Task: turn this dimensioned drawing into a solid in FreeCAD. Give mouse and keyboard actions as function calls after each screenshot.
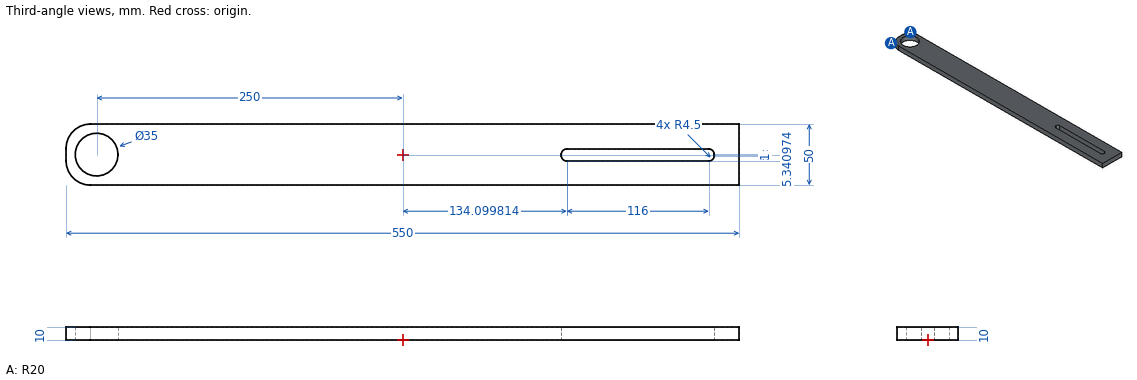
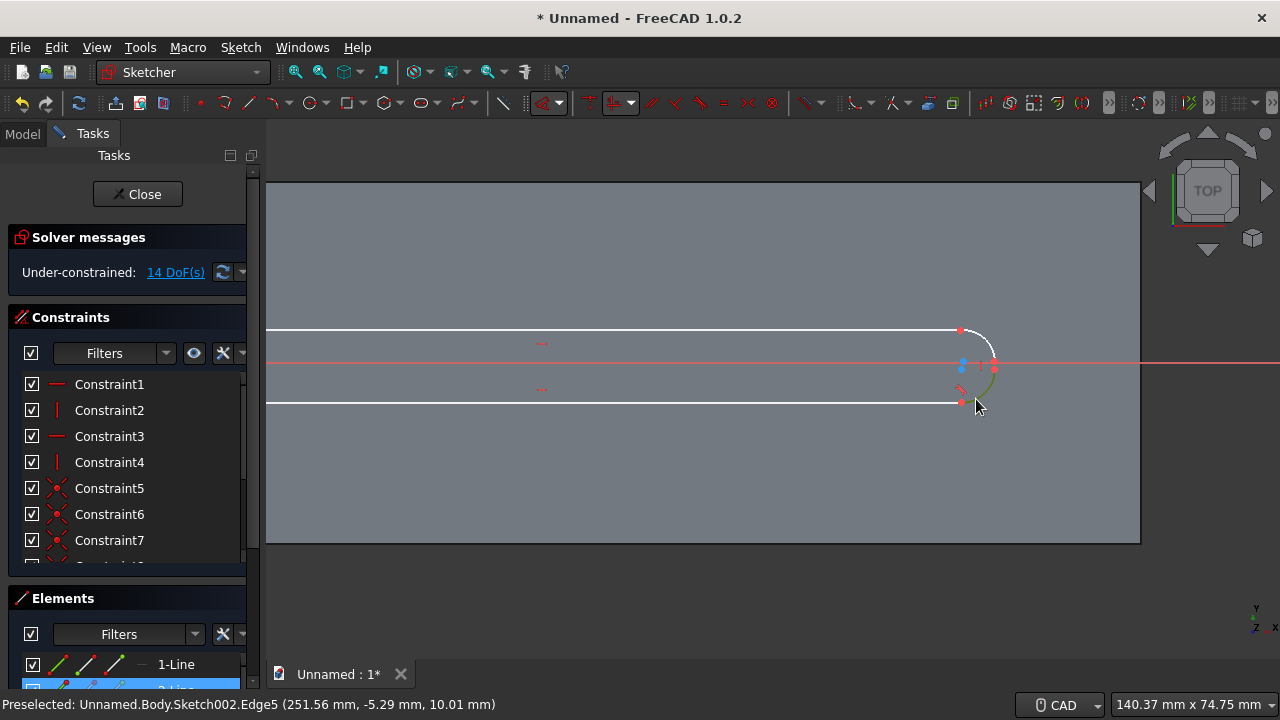
click(700, 104)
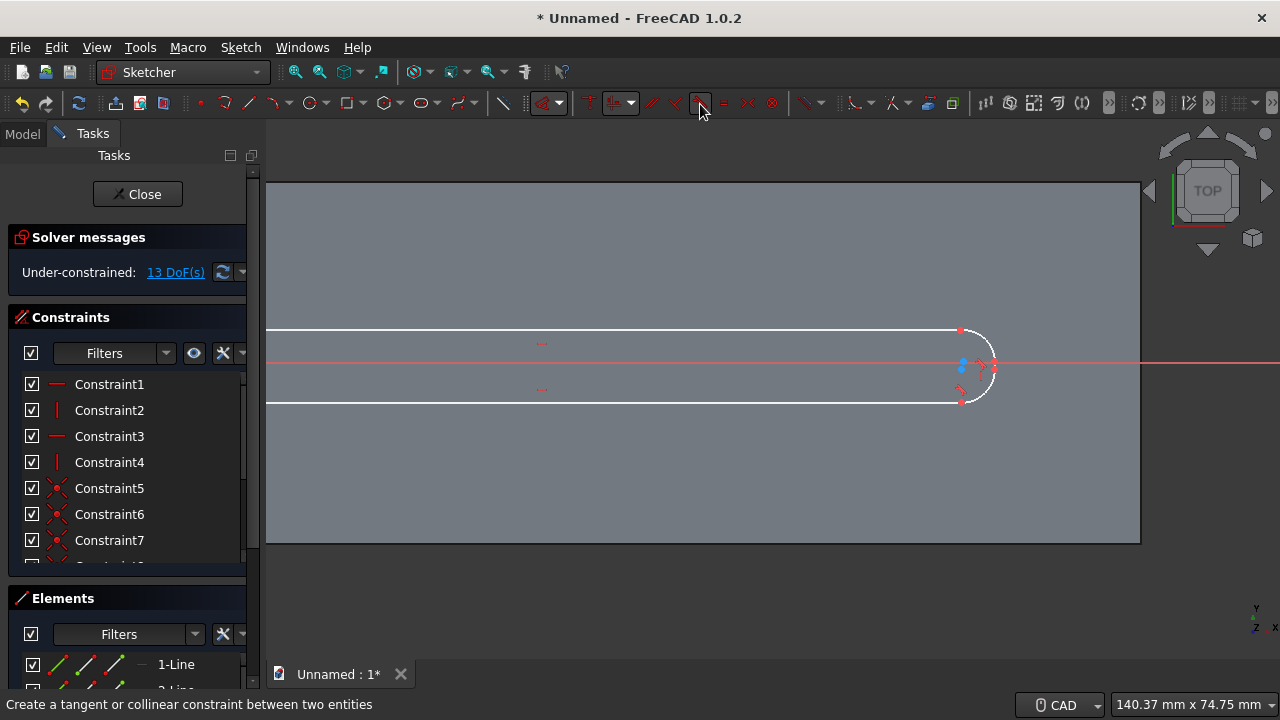
scroll(995, 366, up, 7)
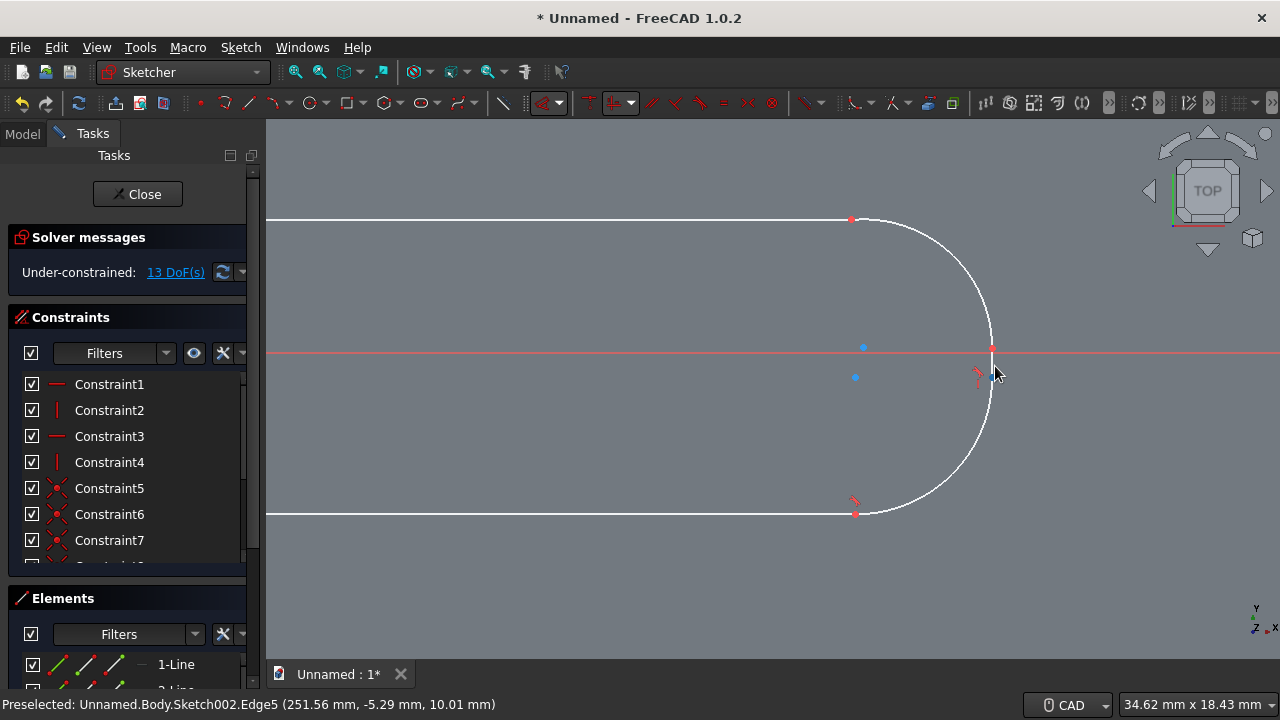
click(992, 363)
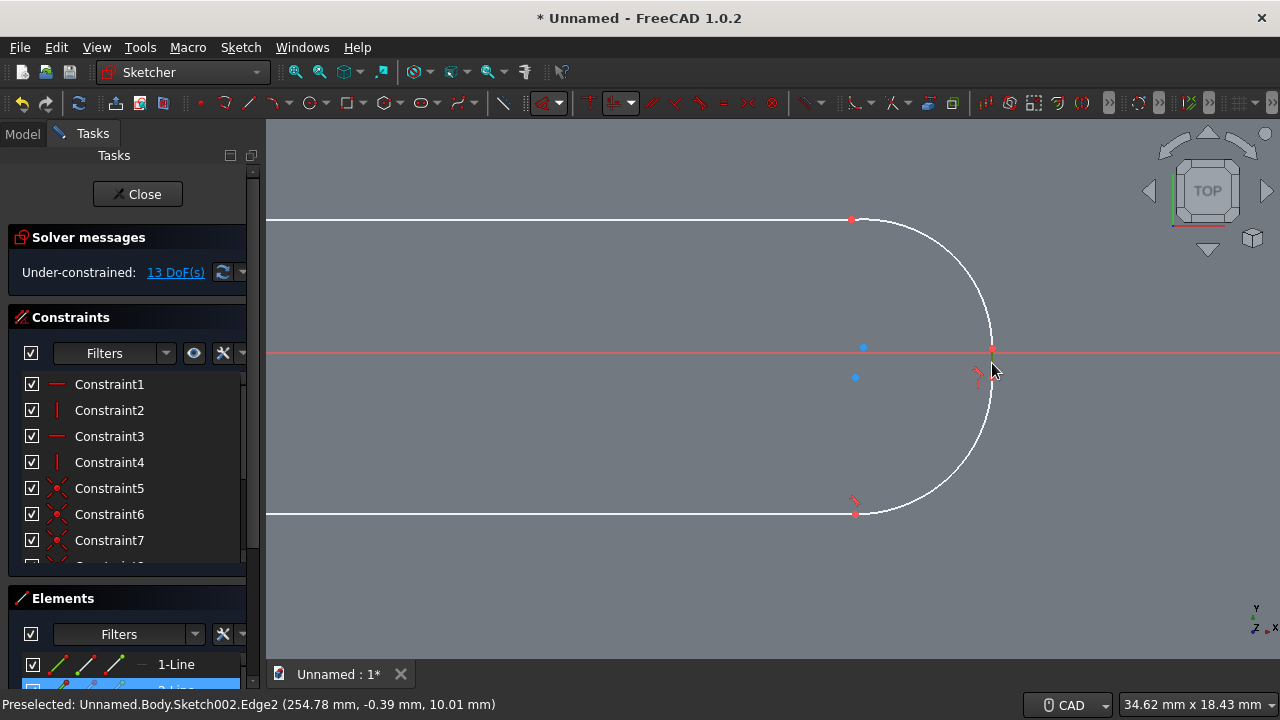
scroll(981, 391, down, 13)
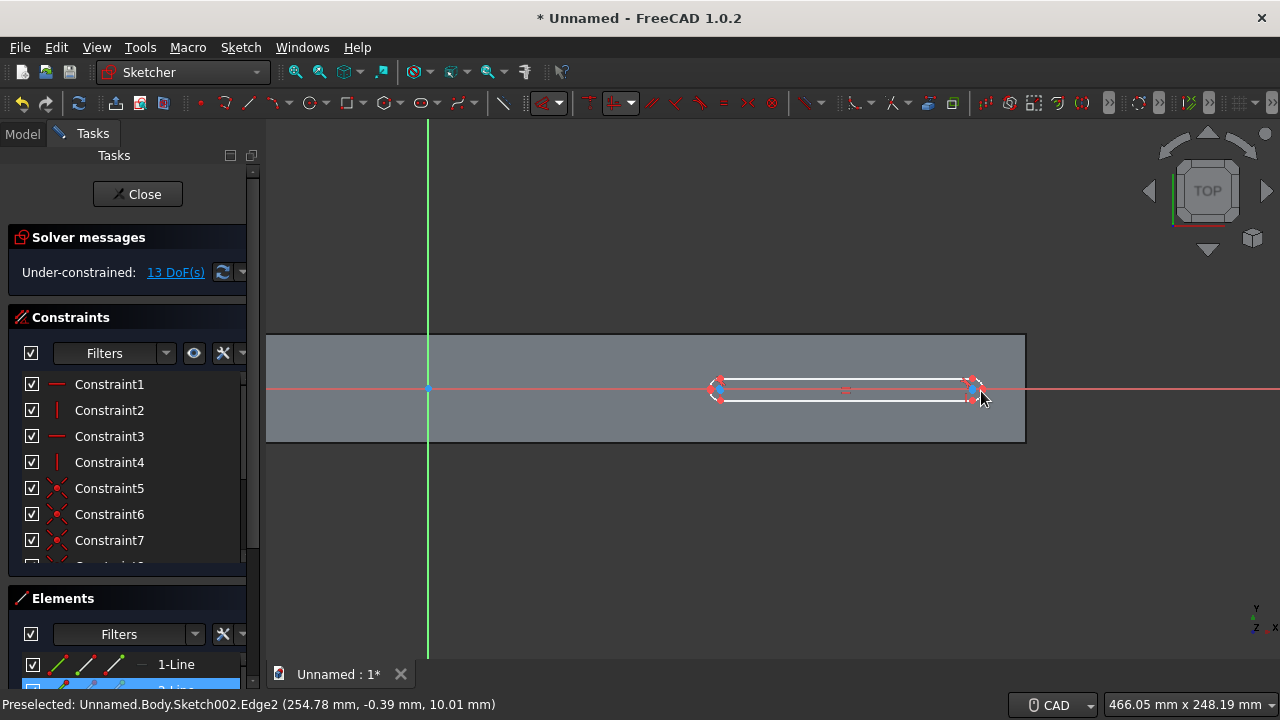
scroll(981, 384, up, 6)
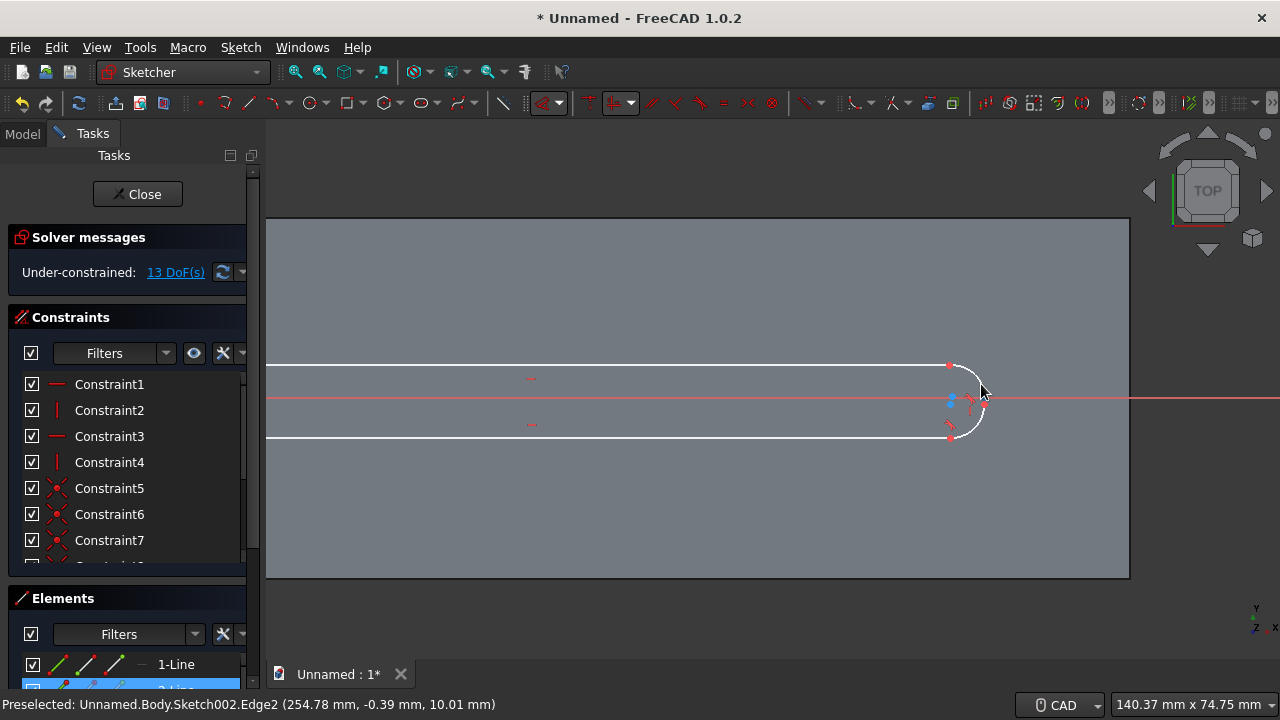
click(980, 382)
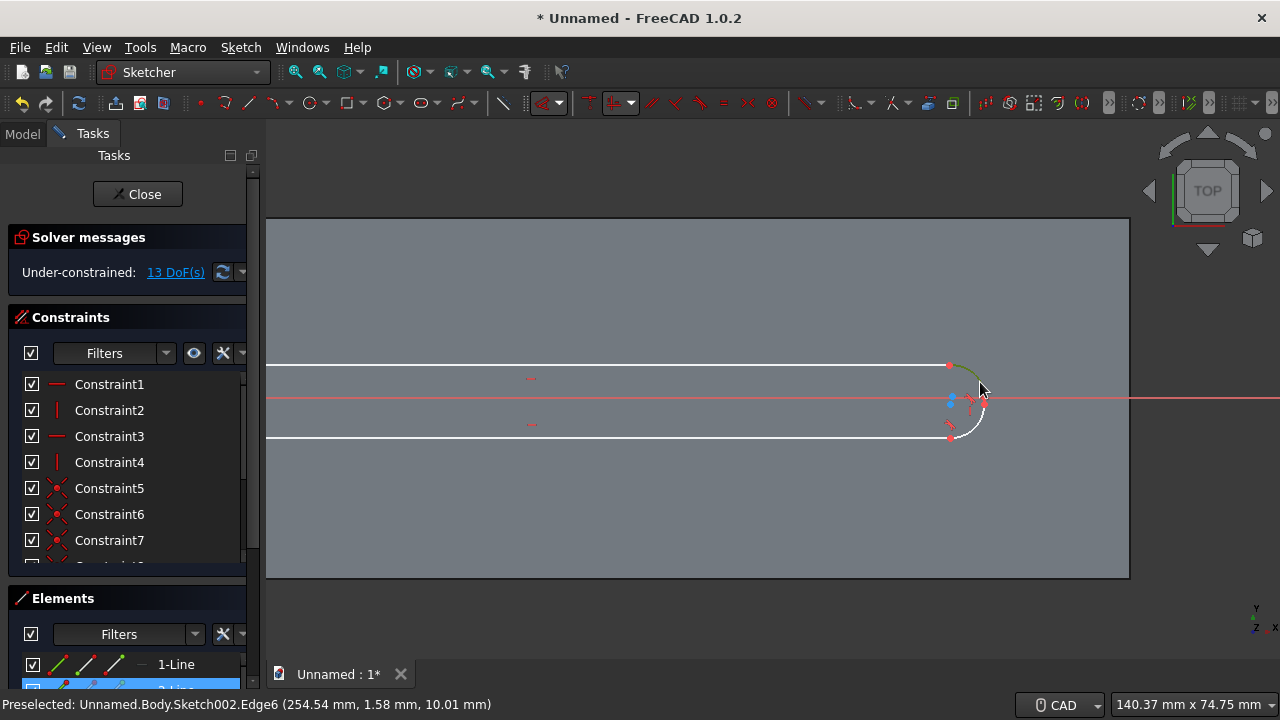
click(700, 104)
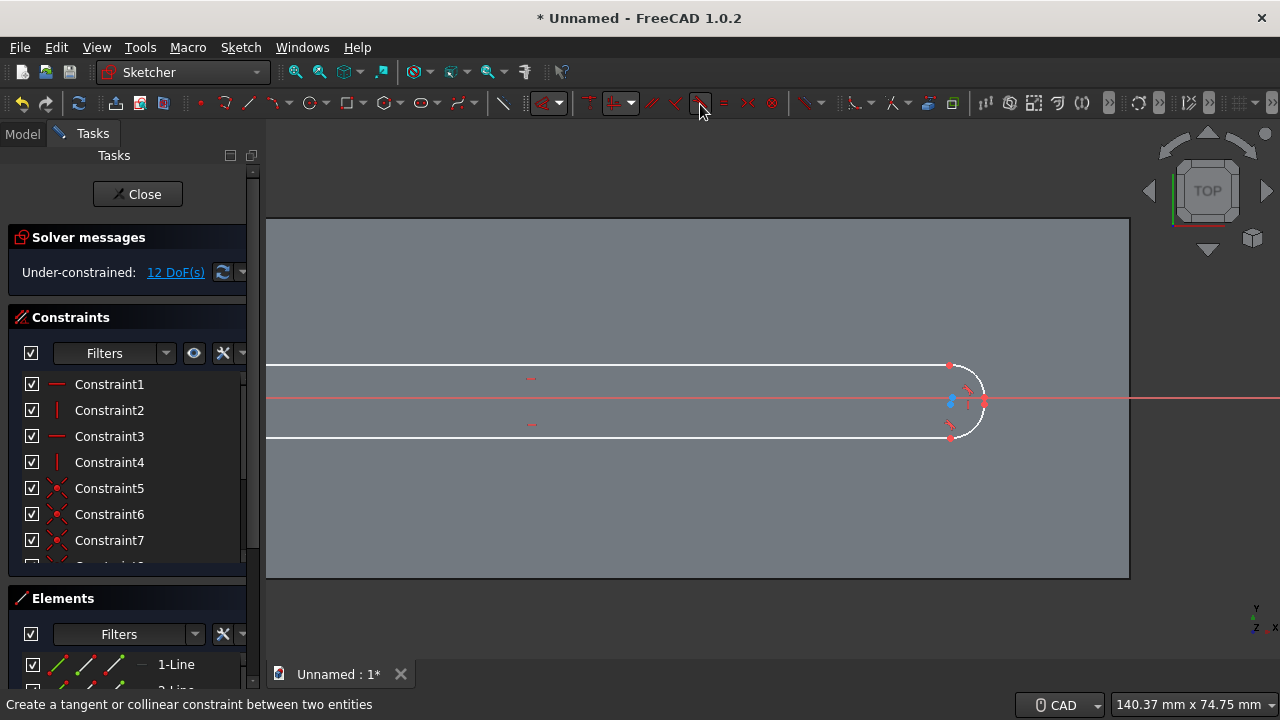
click(699, 365)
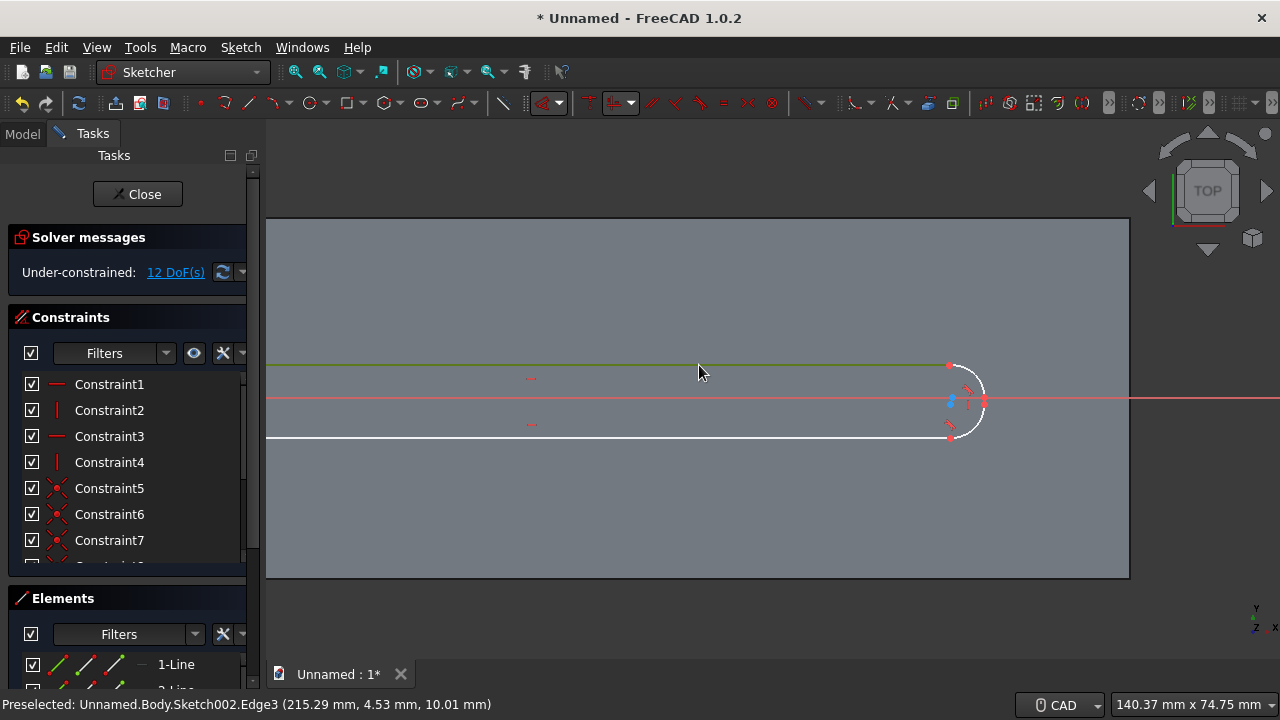
click(980, 382)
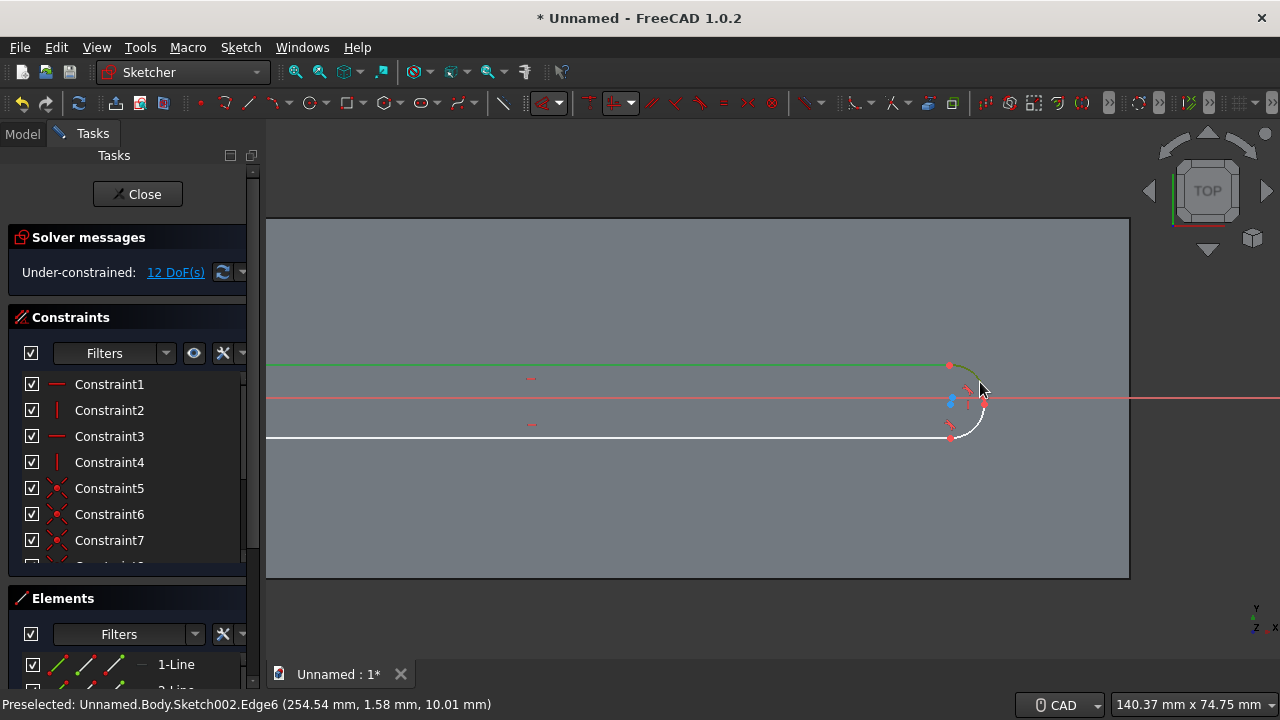
click(700, 104)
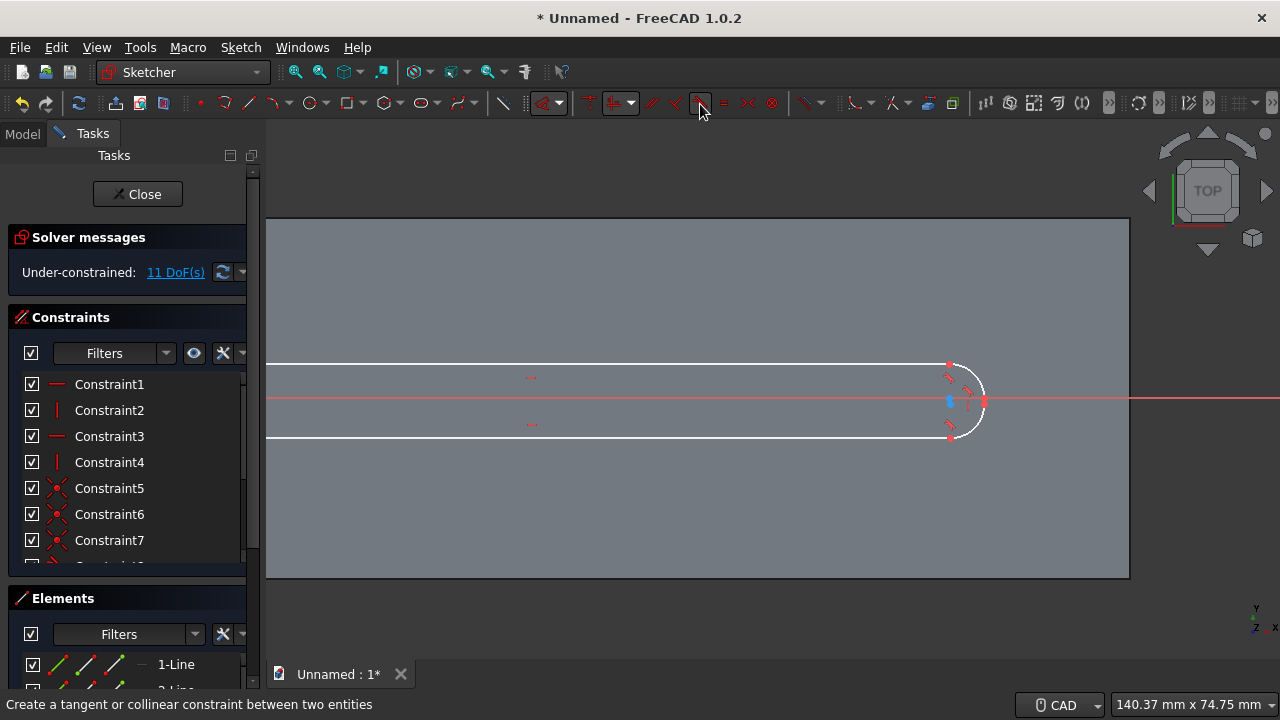
click(699, 364)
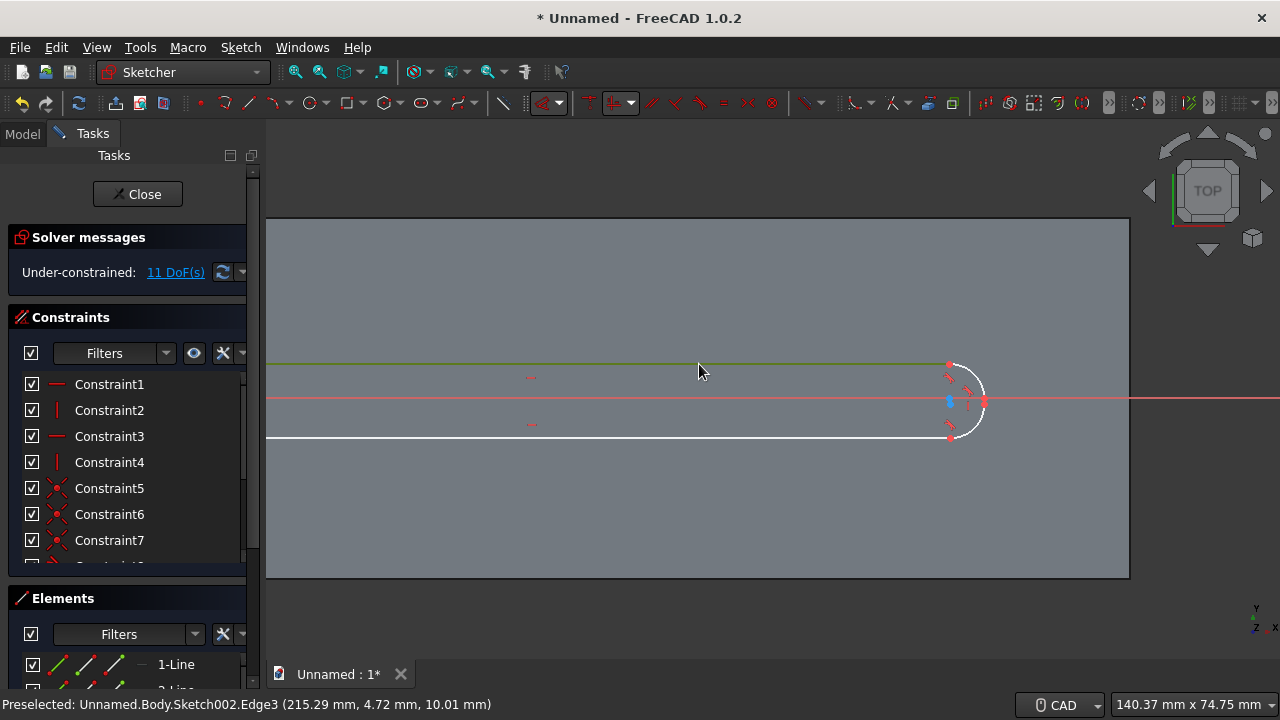
scroll(981, 384, down, 6)